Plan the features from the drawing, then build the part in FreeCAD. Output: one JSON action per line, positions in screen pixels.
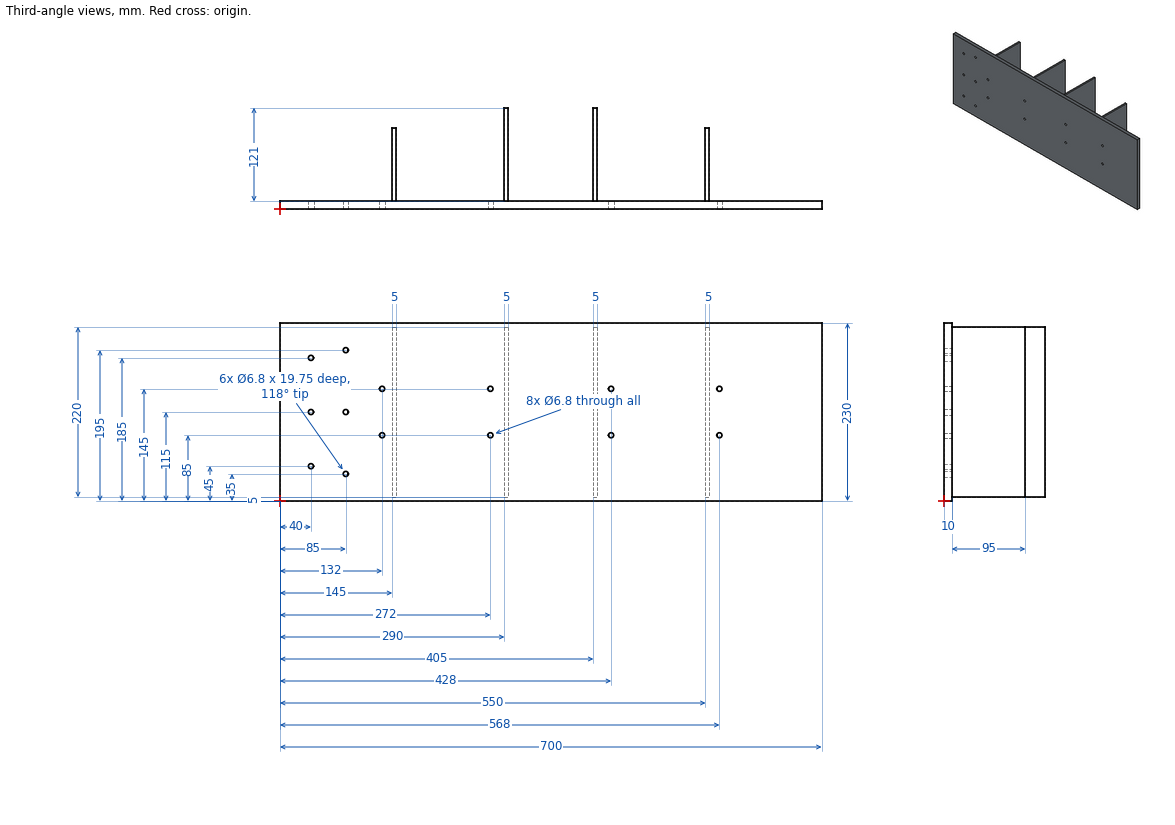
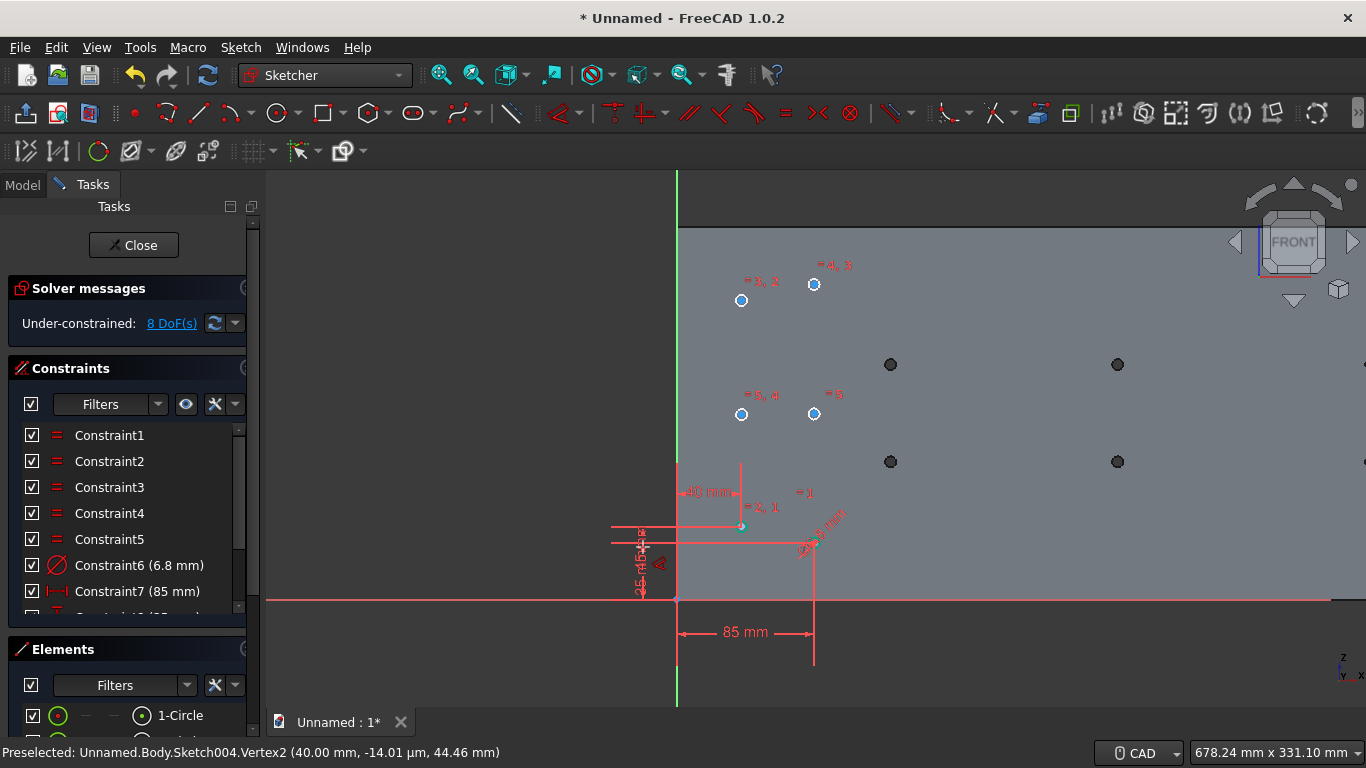
{"action": "left_click", "coordinate": [742, 300]}
{"action": "left_click", "coordinate": [709, 266]}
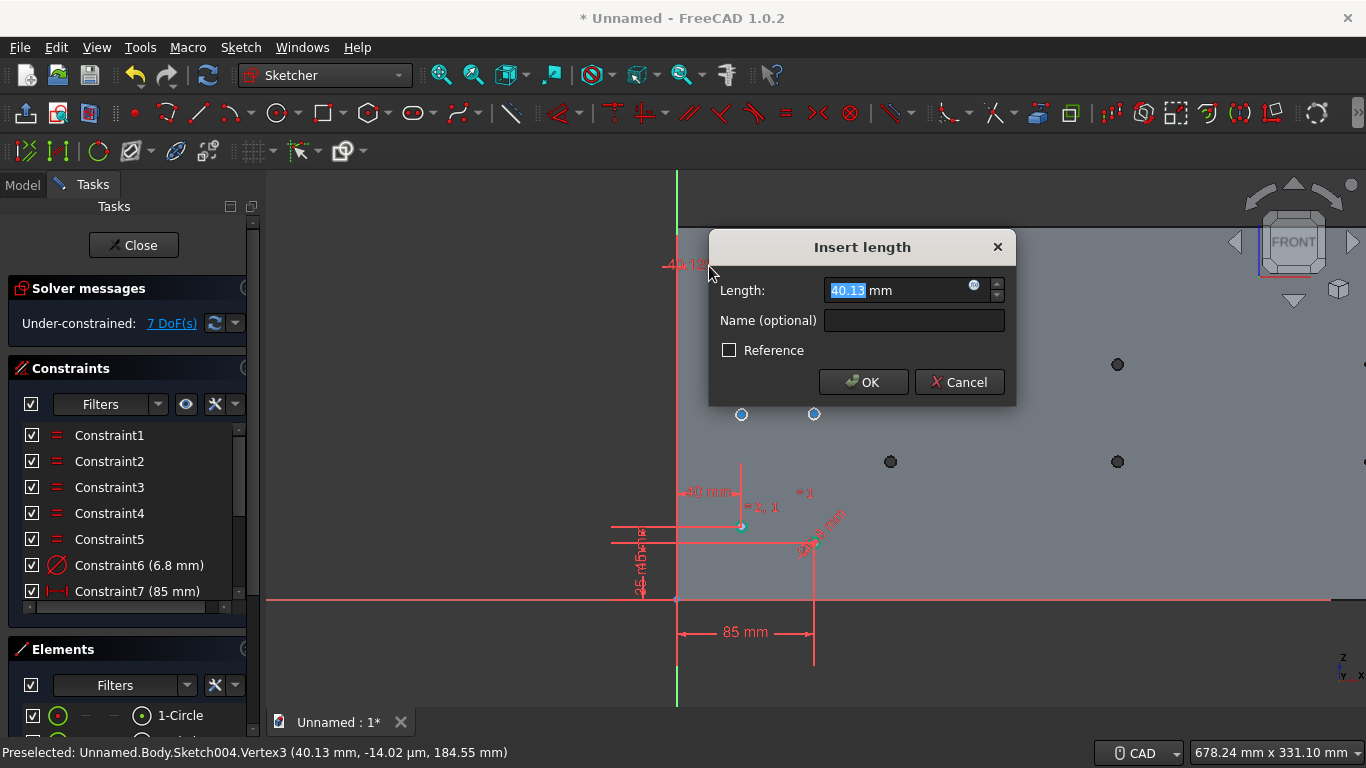
{"action": "type", "text": "40"}
{"action": "key", "text": "Return"}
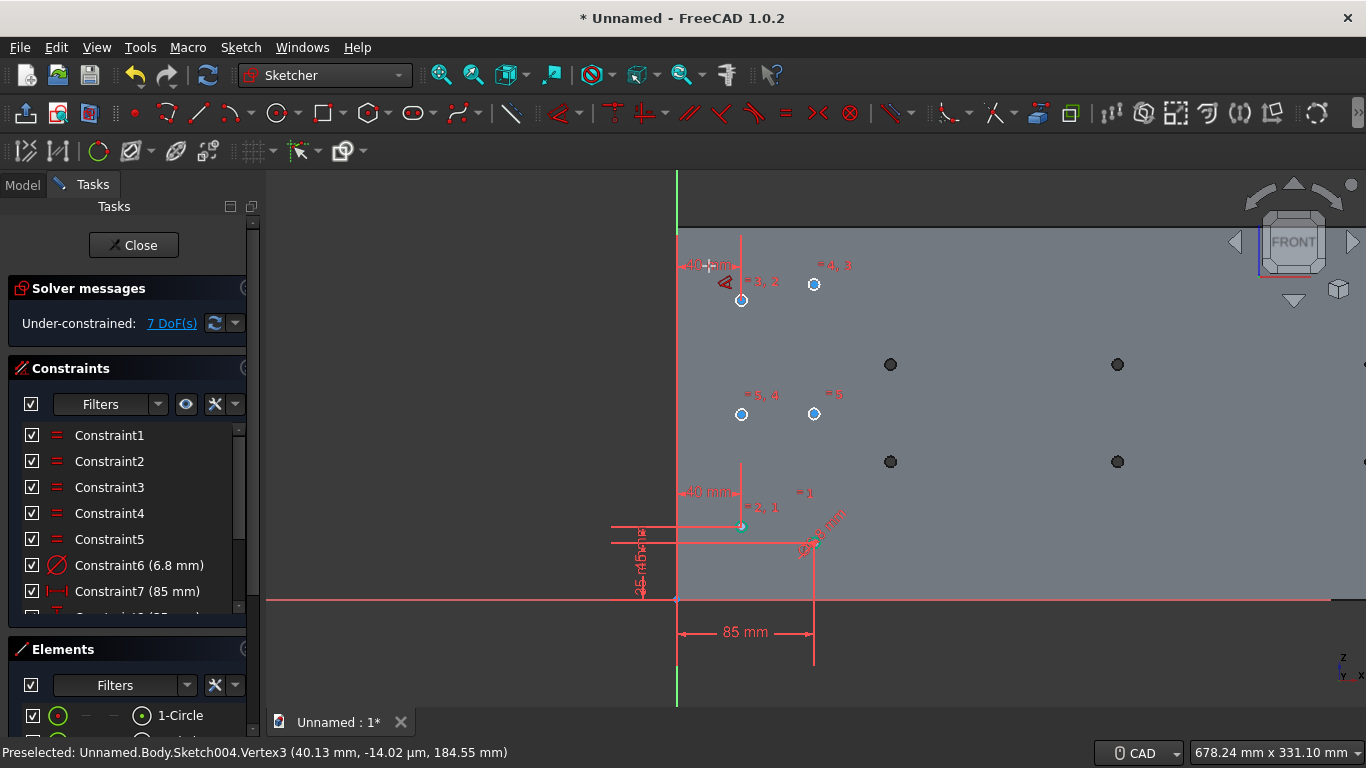
{"action": "left_click", "coordinate": [814, 285]}
{"action": "left_click", "coordinate": [793, 251]}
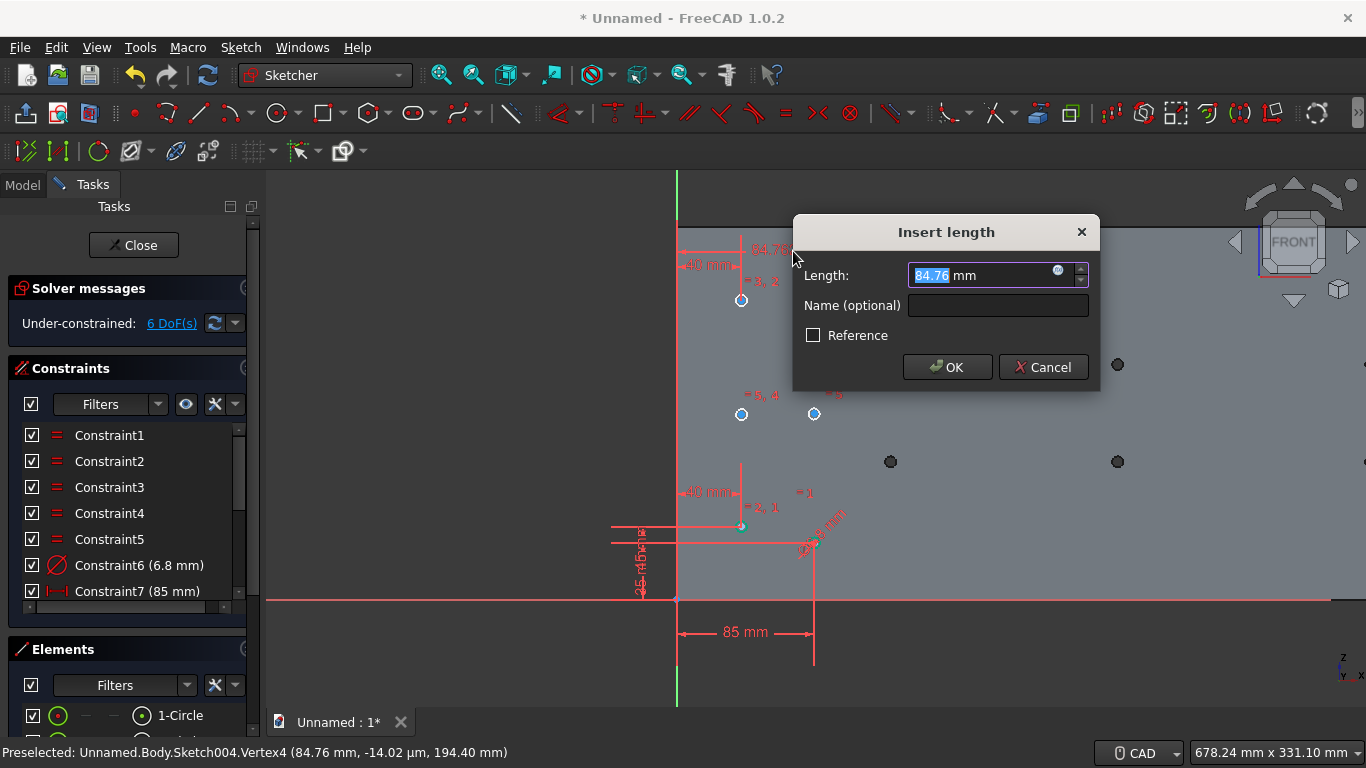
{"action": "type", "text": "85"}
{"action": "key", "text": "Return"}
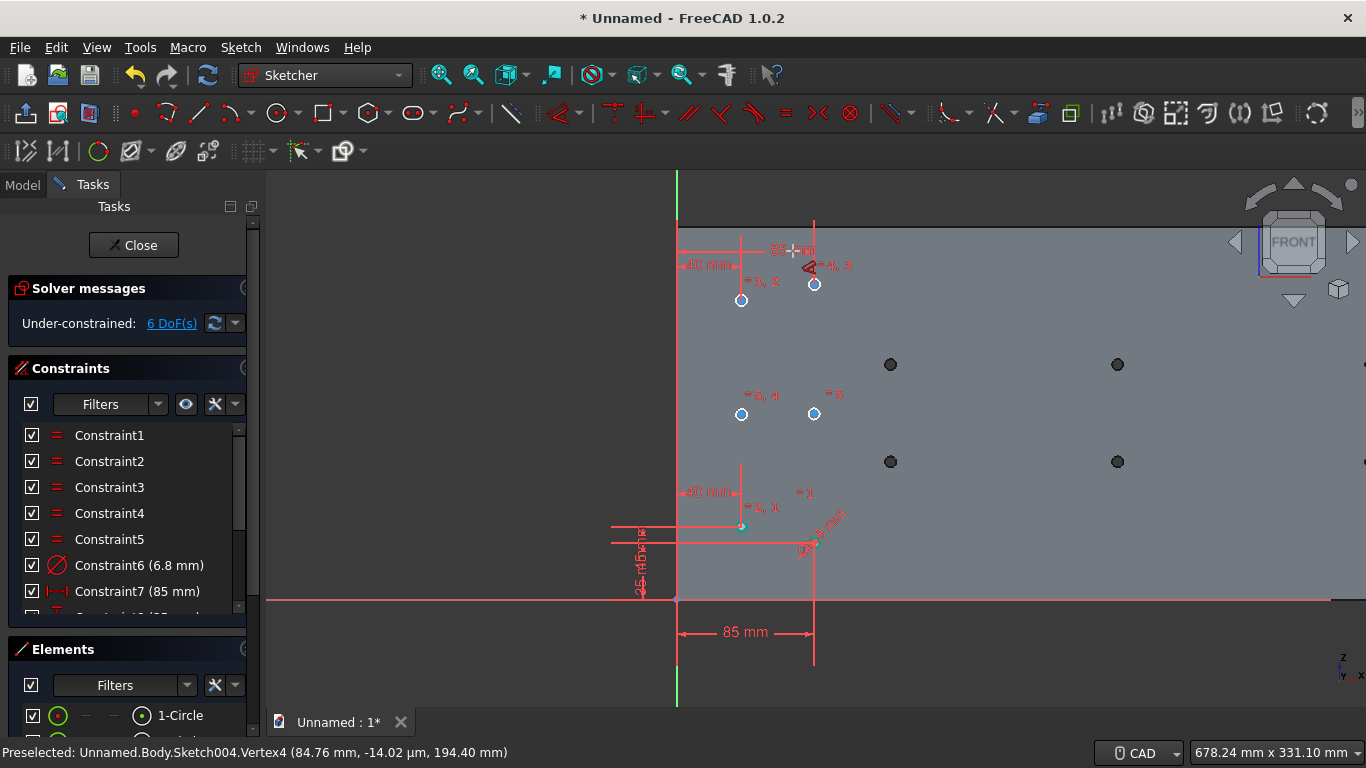
{"action": "left_click", "coordinate": [742, 415]}
{"action": "left_click", "coordinate": [709, 381]}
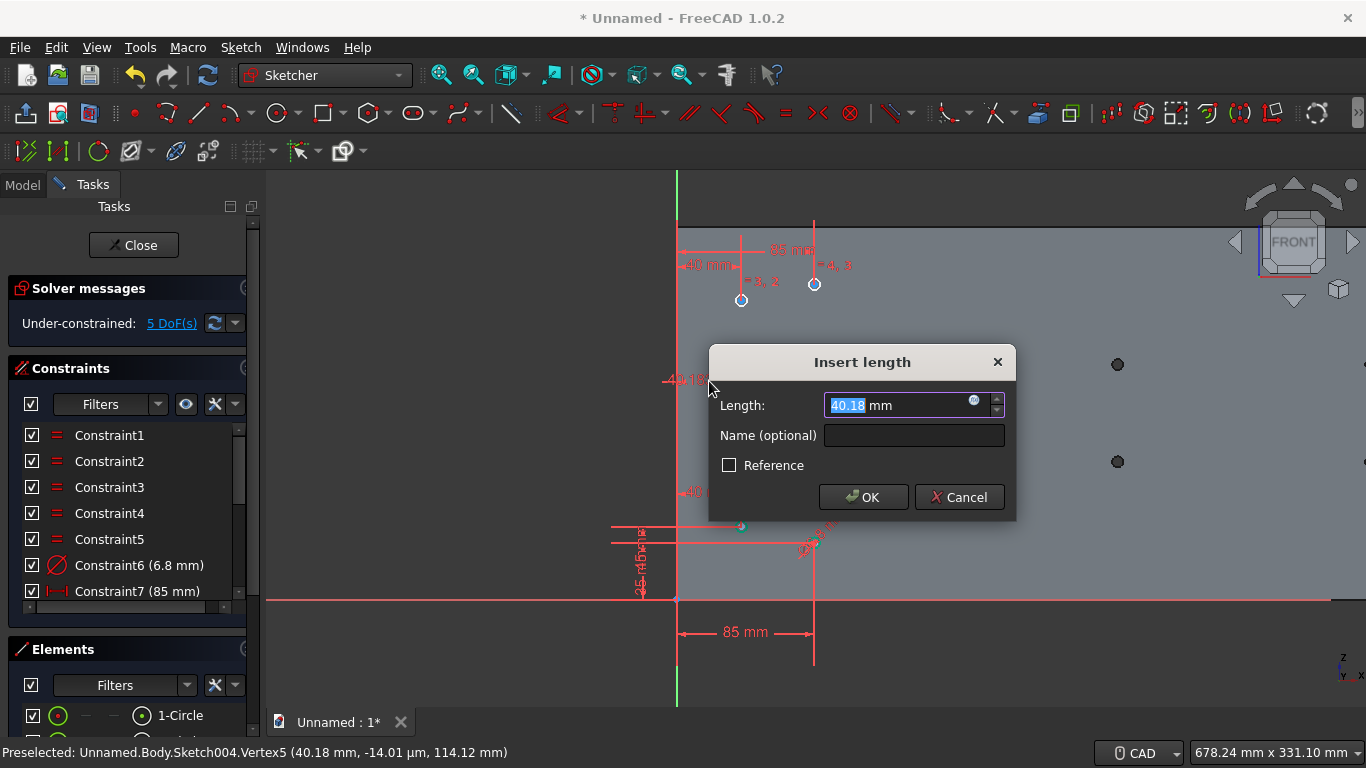
{"action": "type", "text": "40"}
{"action": "key", "text": "Return"}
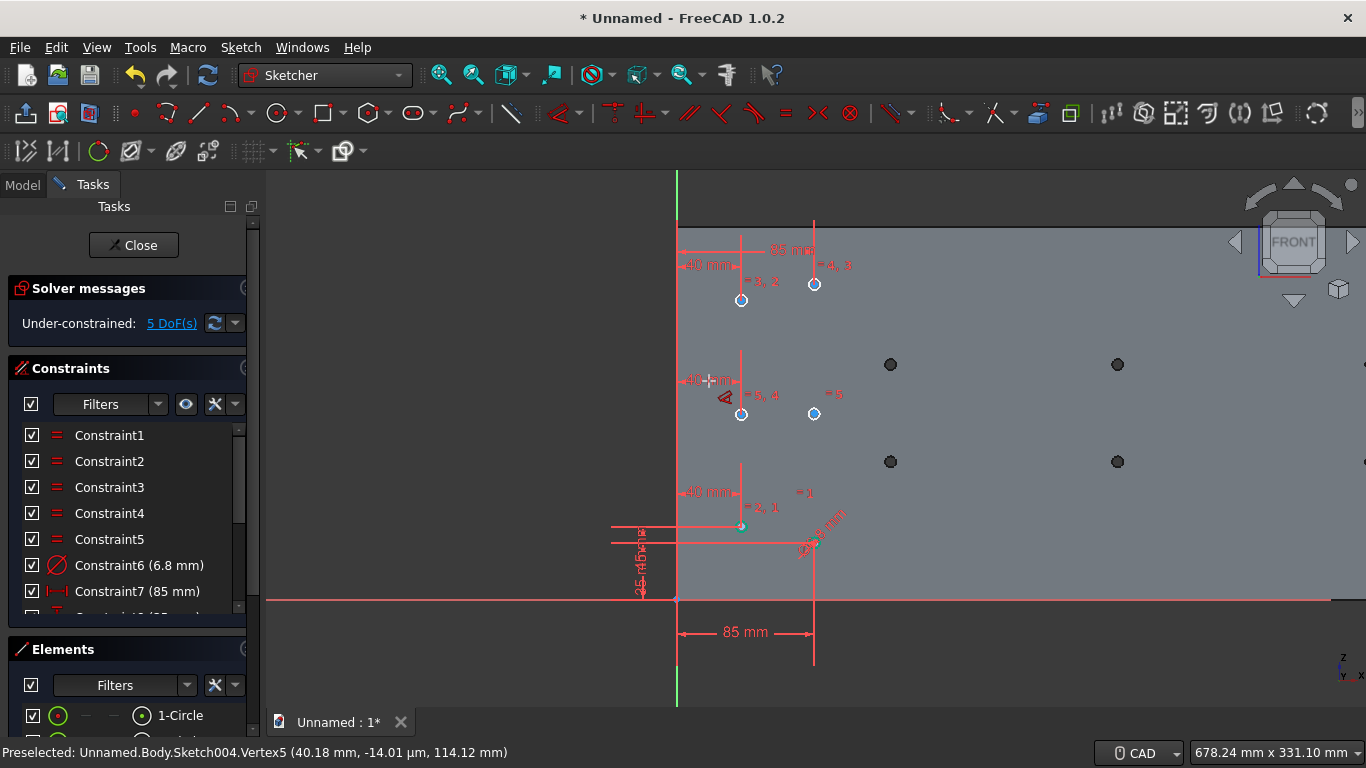
{"action": "left_click", "coordinate": [814, 414]}
{"action": "left_click", "coordinate": [793, 380]}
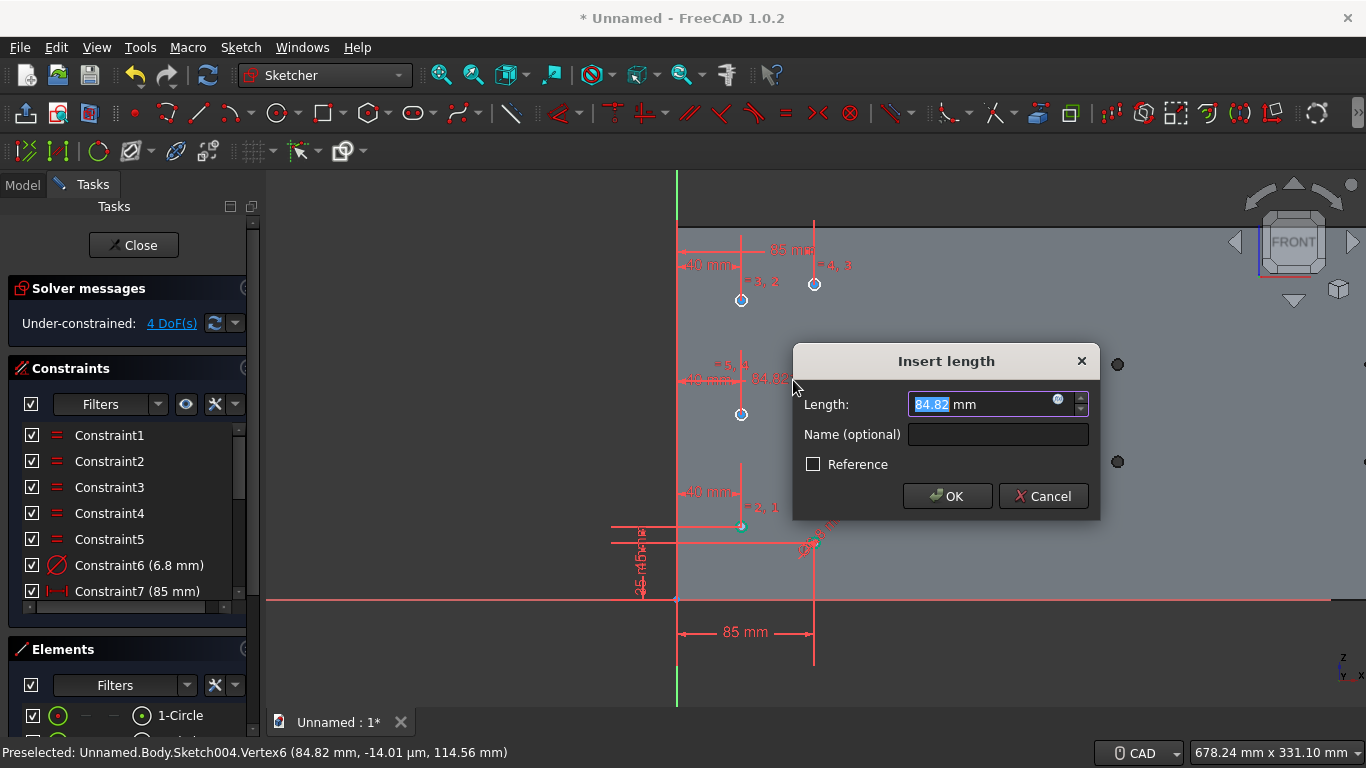
{"action": "type", "text": "85"}
{"action": "key", "text": "Return"}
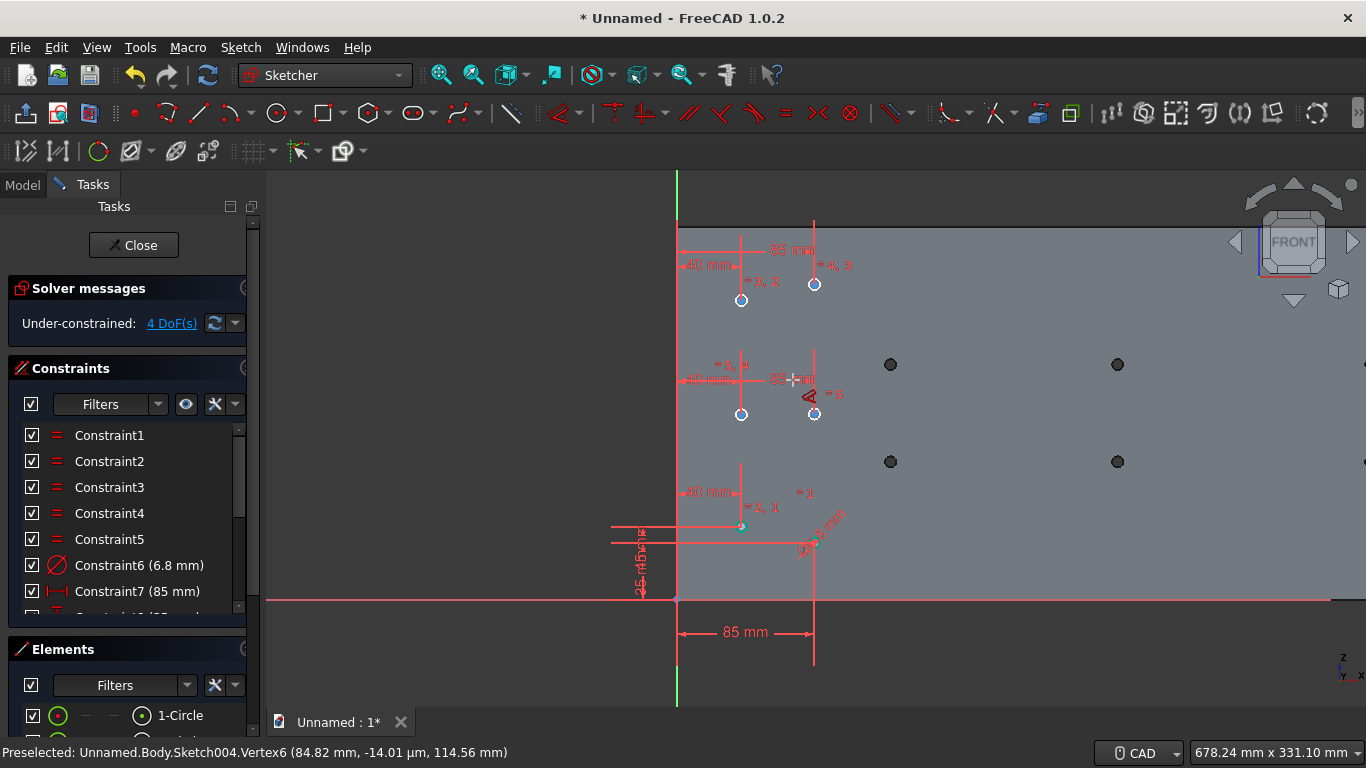
{"action": "left_click", "coordinate": [741, 300]}
{"action": "left_click", "coordinate": [643, 450]}